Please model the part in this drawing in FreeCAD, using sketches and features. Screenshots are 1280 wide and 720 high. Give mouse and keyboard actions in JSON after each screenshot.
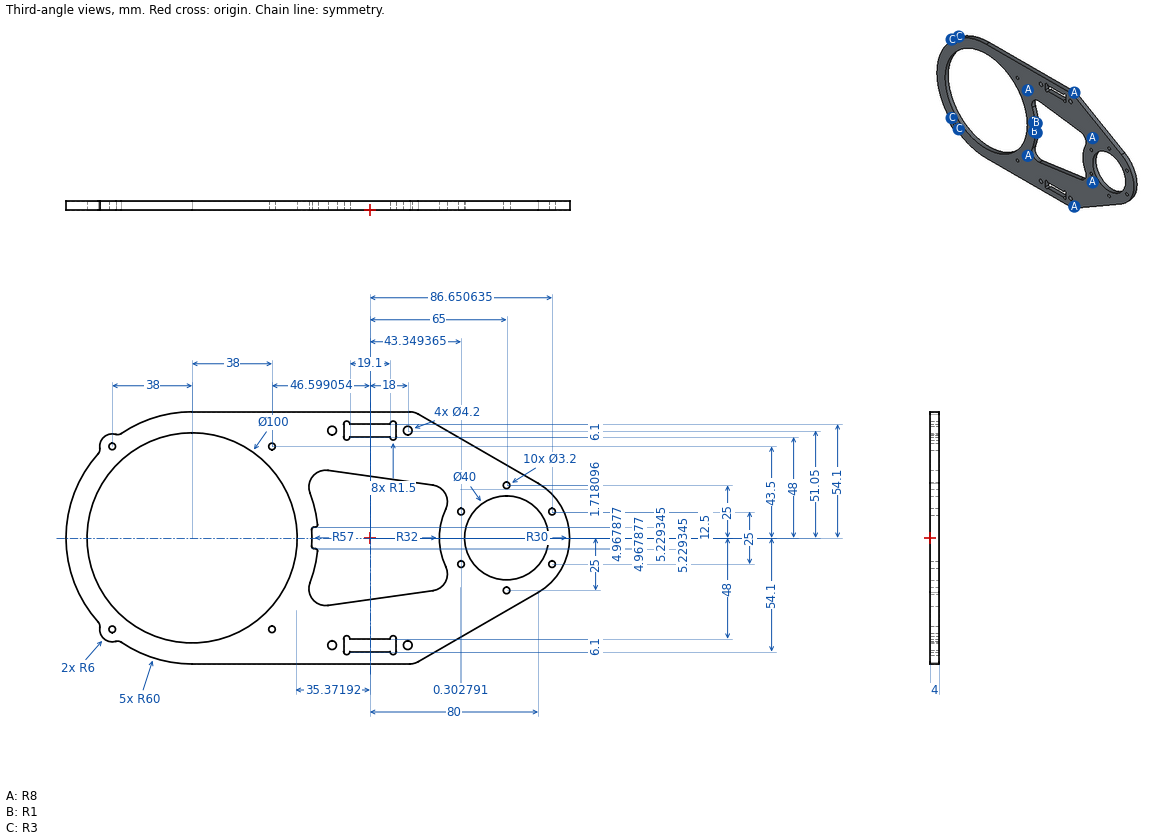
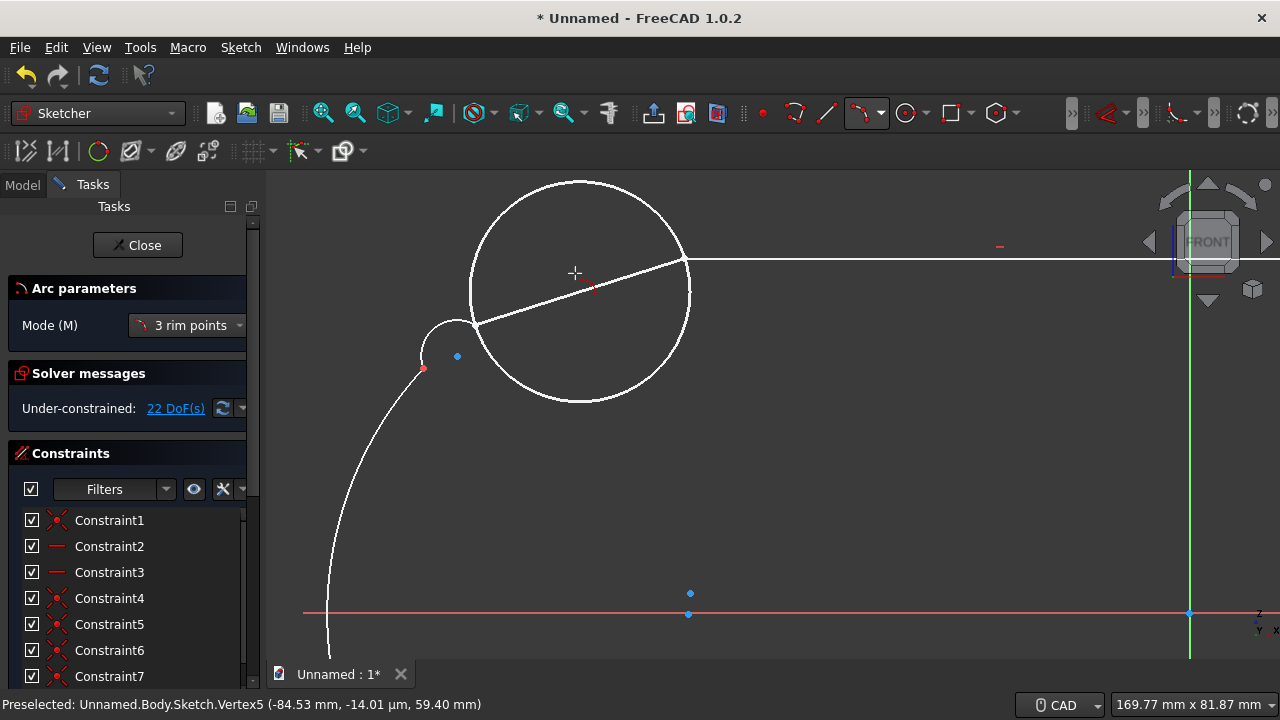
{"action": "left_click", "coordinate": [575, 272]}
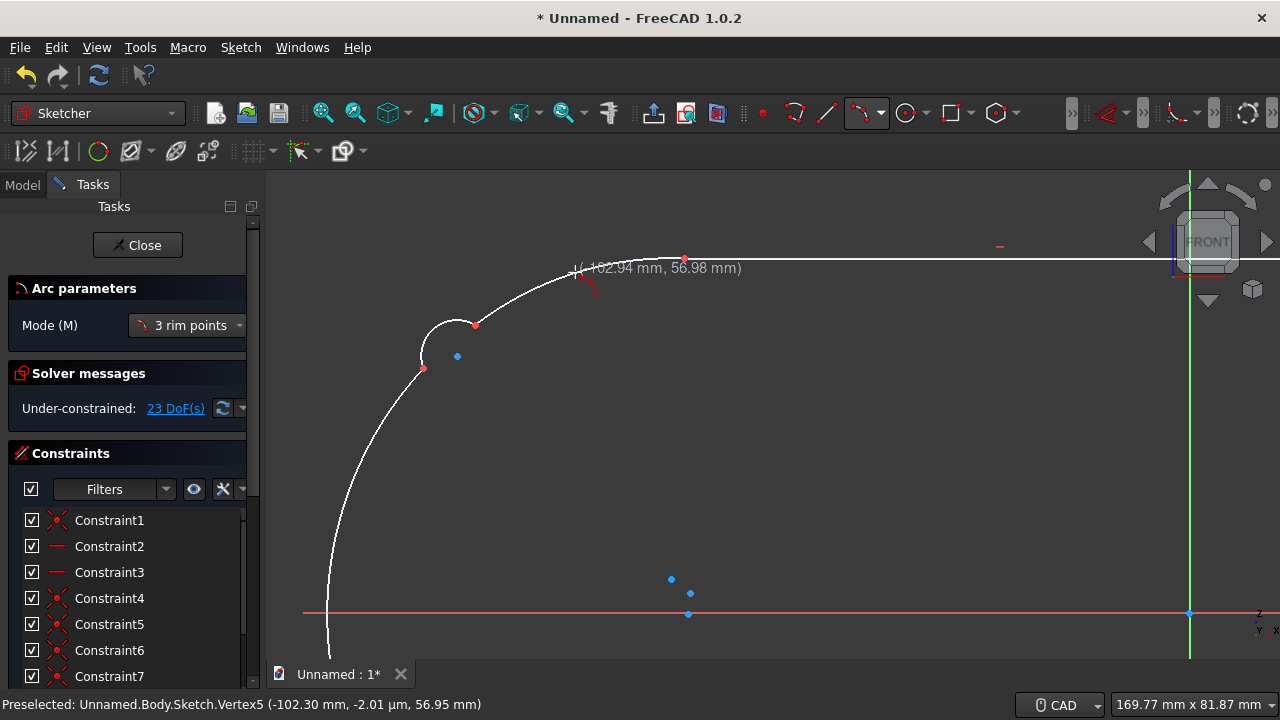
{"action": "scroll", "coordinate": [508, 299], "scroll_direction": "down", "scroll_amount": 5}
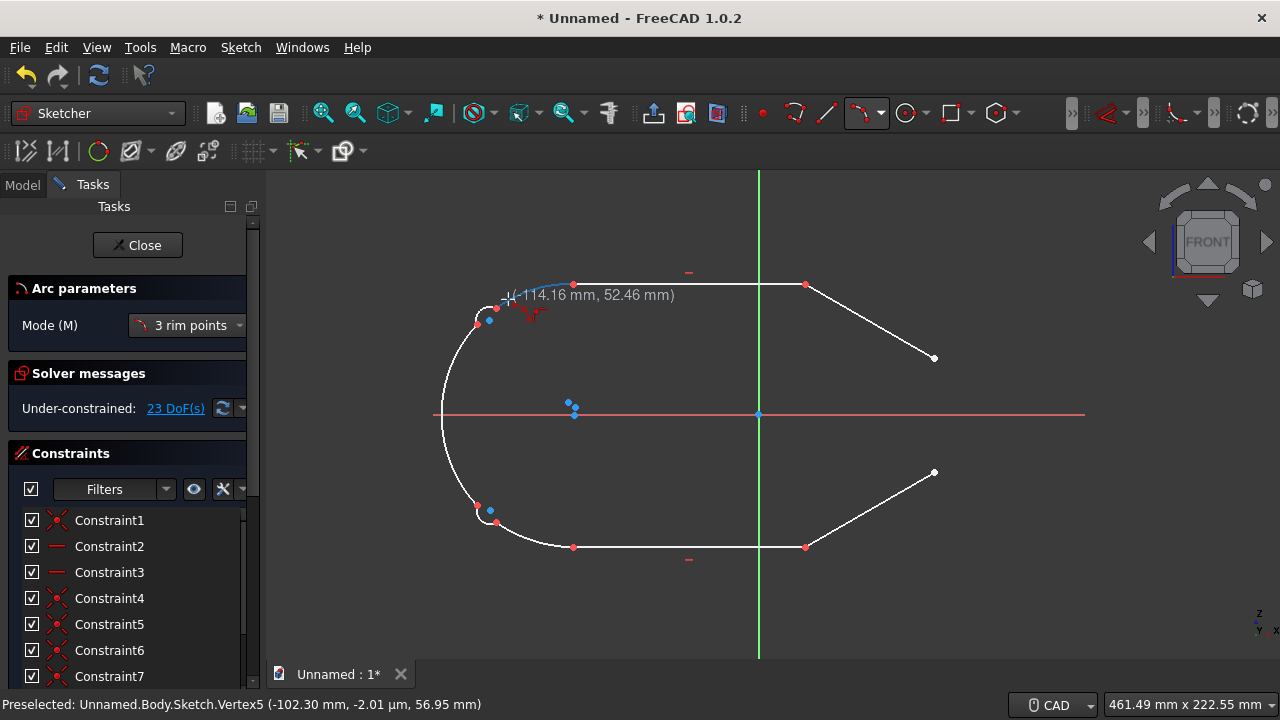
{"action": "left_click", "coordinate": [935, 359]}
{"action": "left_click", "coordinate": [935, 473]}
{"action": "left_click", "coordinate": [962, 442]}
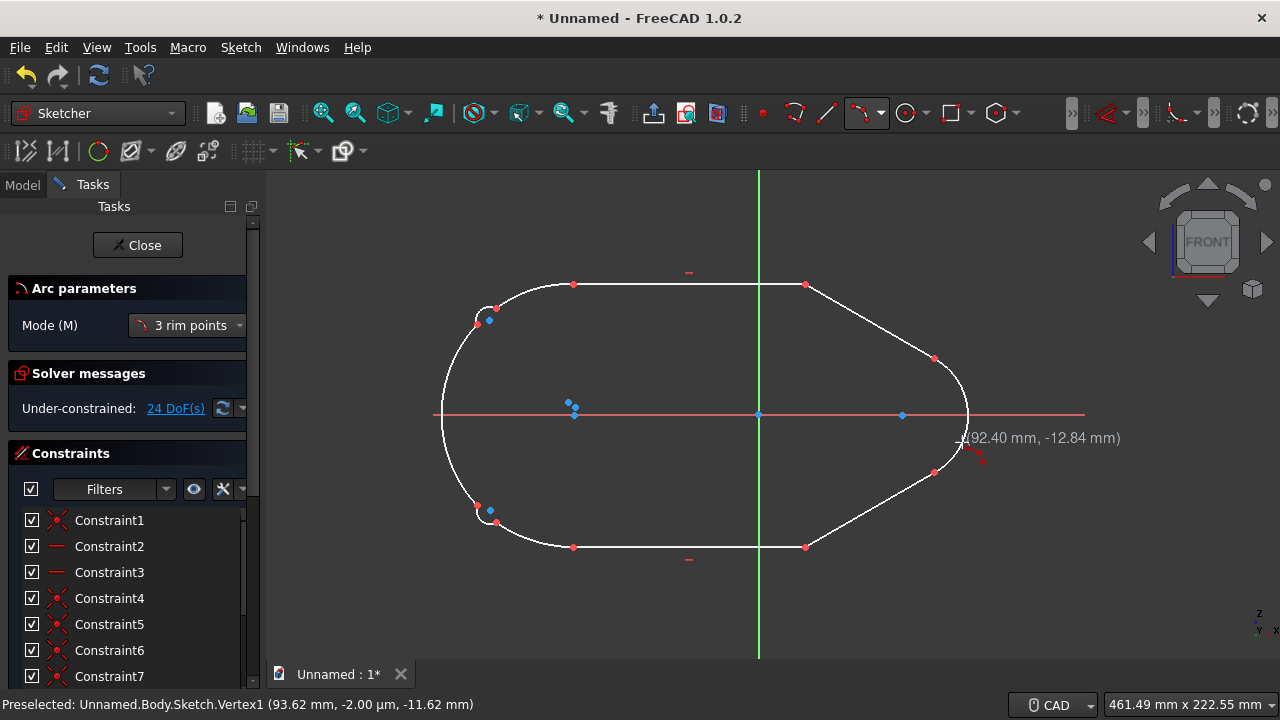
{"action": "key", "text": "g l"}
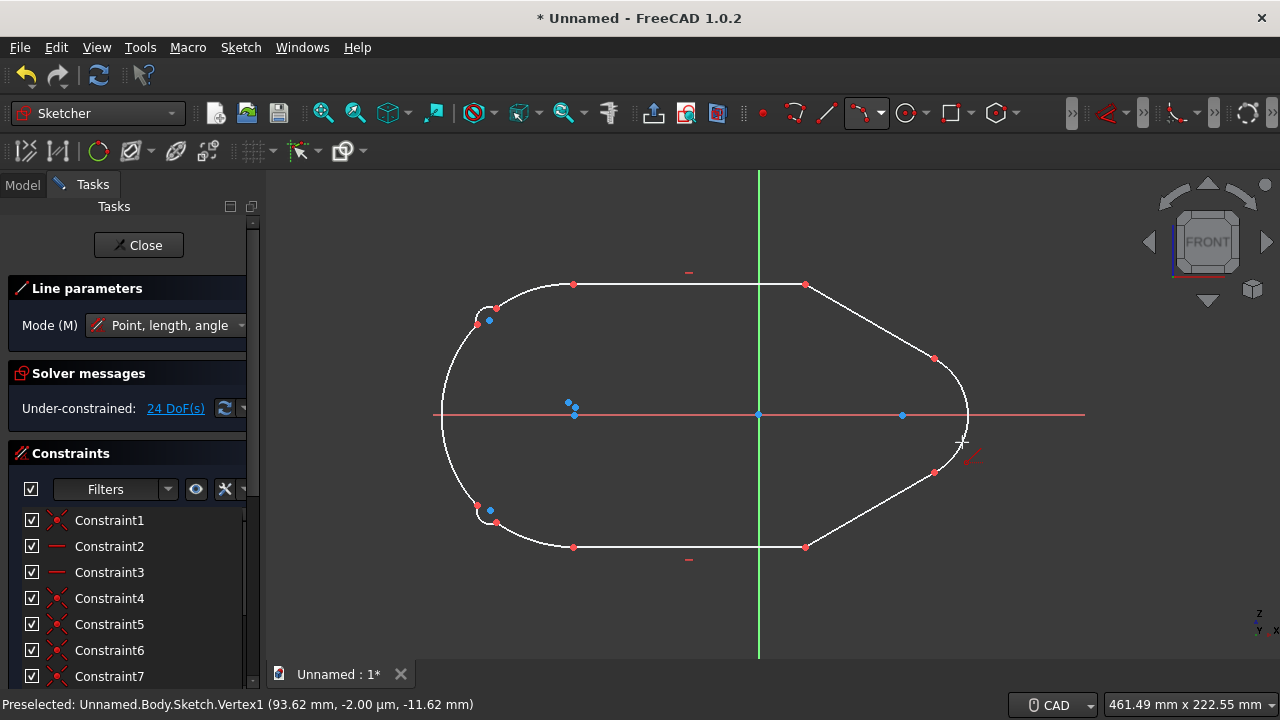
{"action": "left_click", "coordinate": [738, 309]}
{"action": "left_click", "coordinate": [780, 309]}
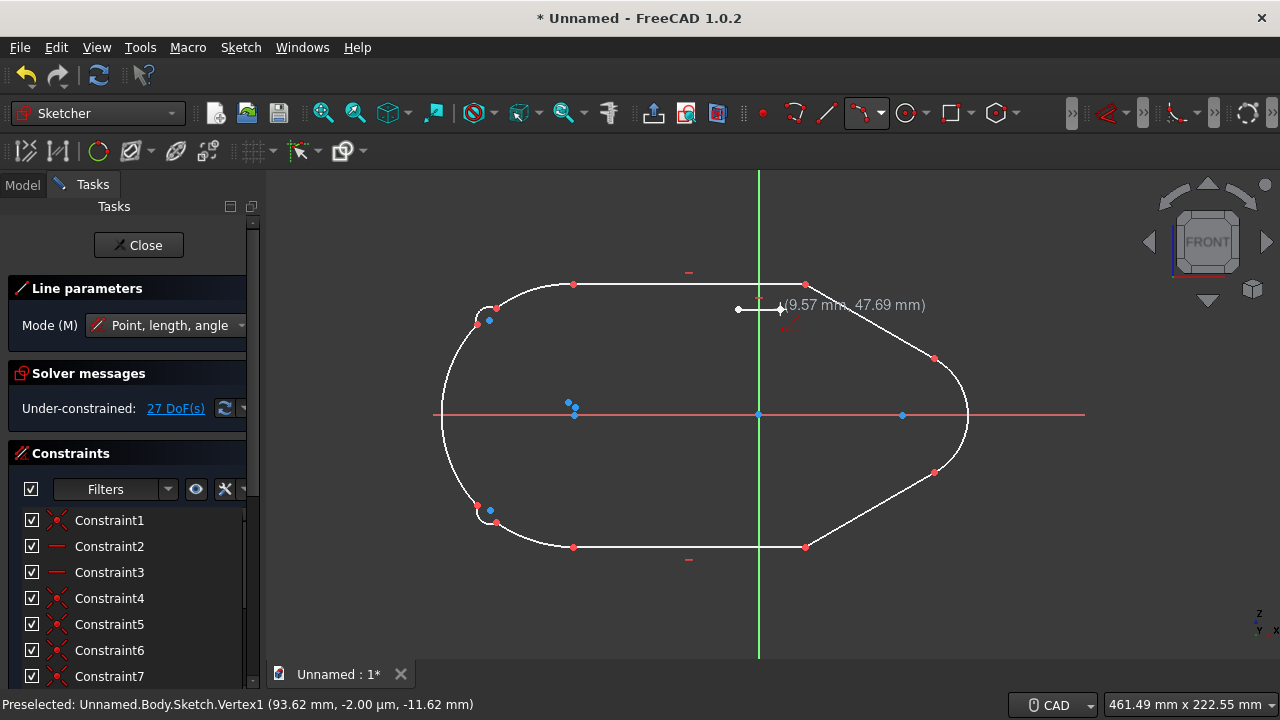
{"action": "scroll", "coordinate": [787, 309], "scroll_direction": "up", "scroll_amount": 5}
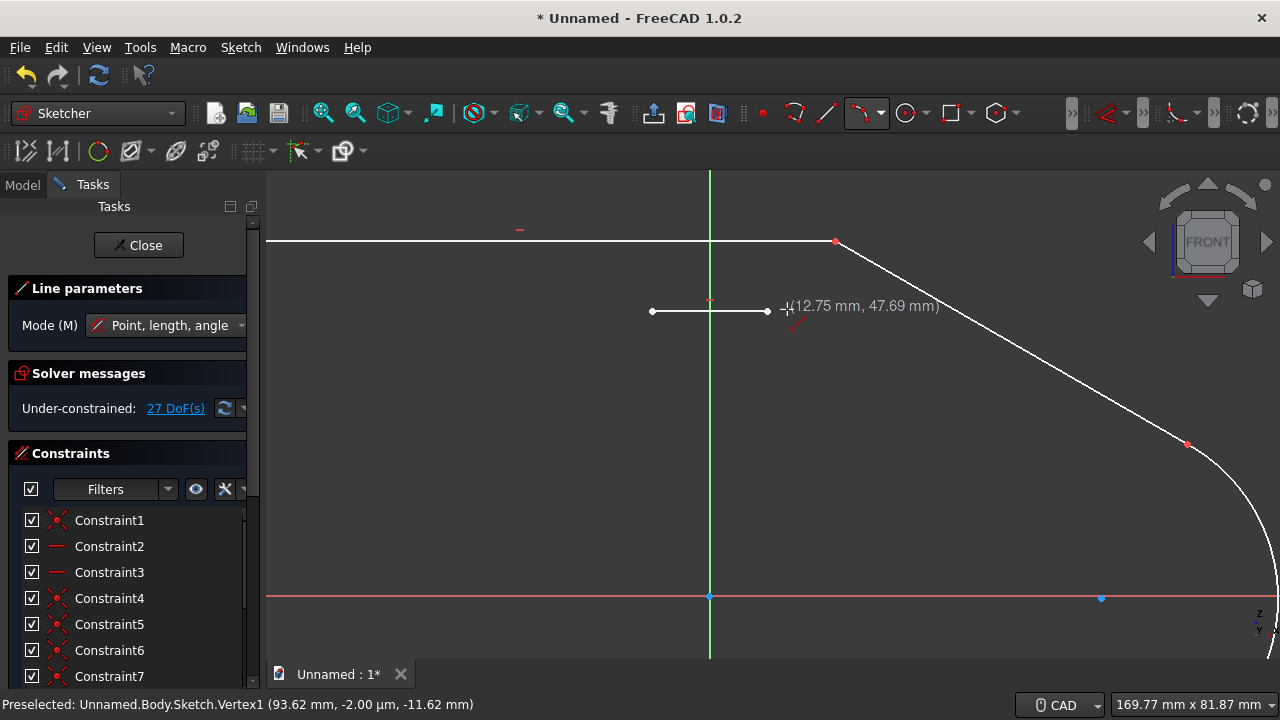
{"action": "left_click", "coordinate": [785, 309]}
{"action": "left_click", "coordinate": [785, 273]}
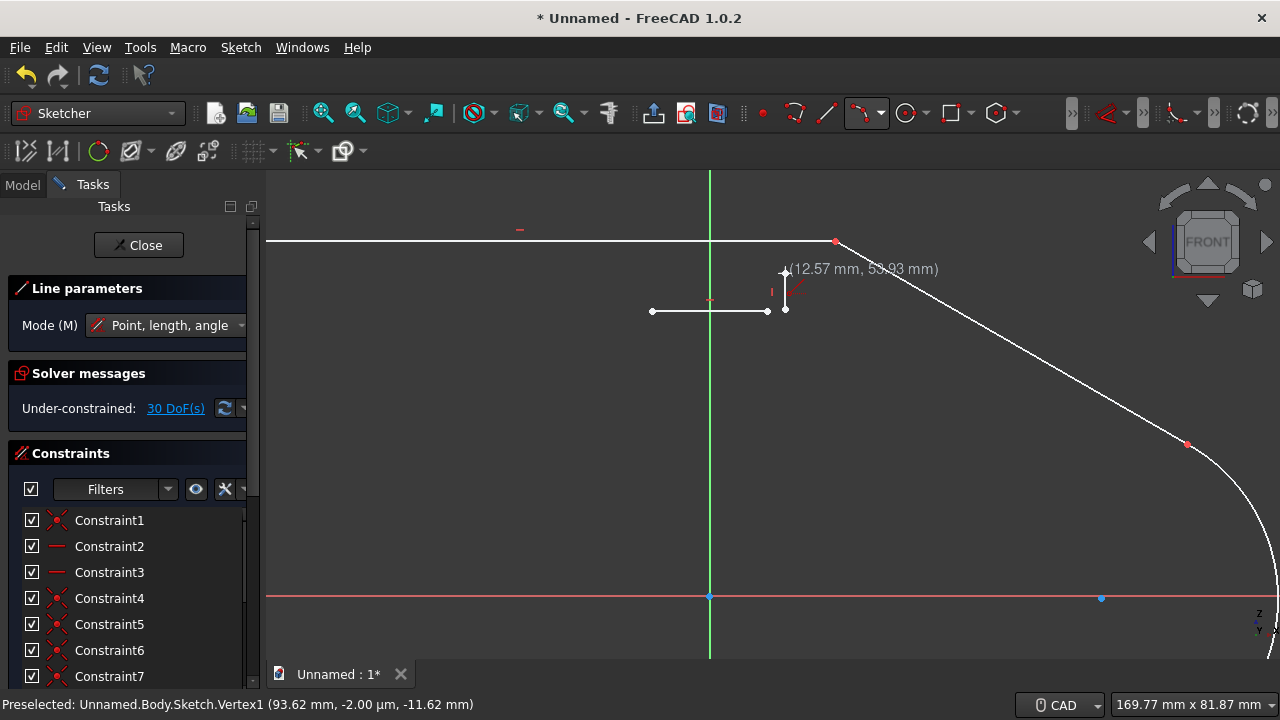
{"action": "left_click", "coordinate": [767, 273]}
{"action": "left_click", "coordinate": [653, 273]}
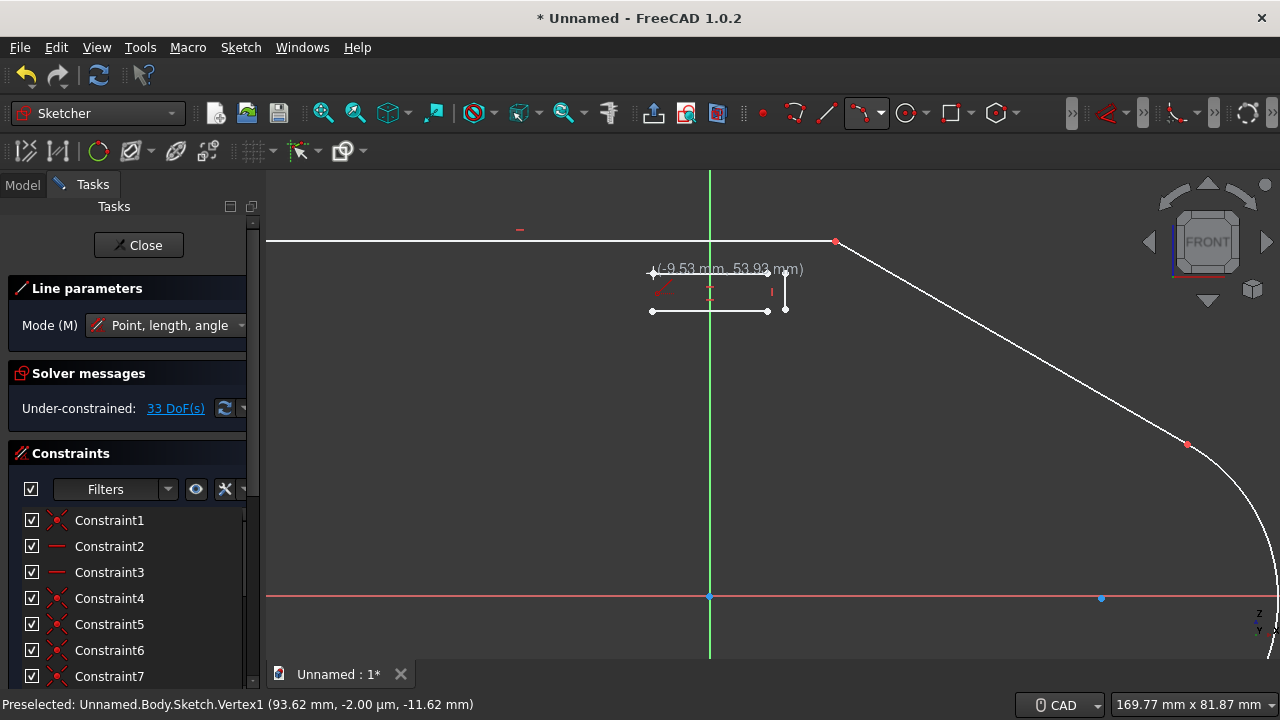
{"action": "left_click", "coordinate": [635, 273]}
{"action": "left_click", "coordinate": [635, 309]}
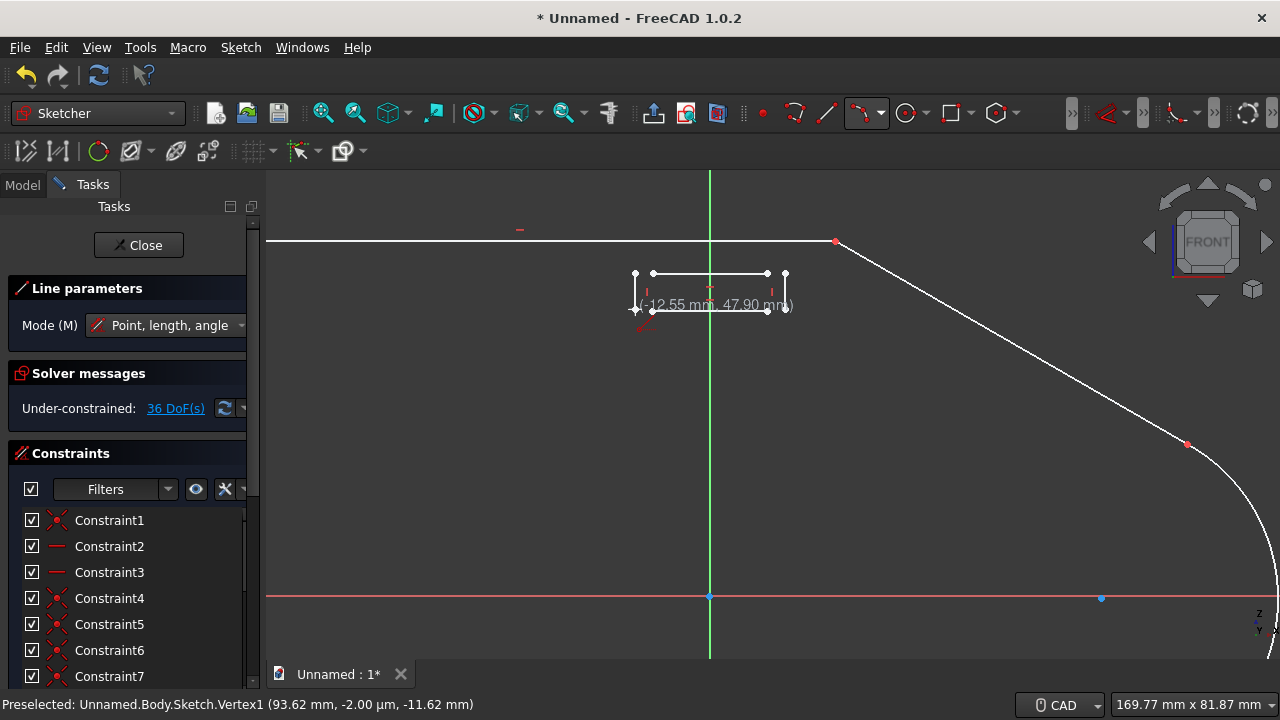
{"action": "key", "text": "g 3 a"}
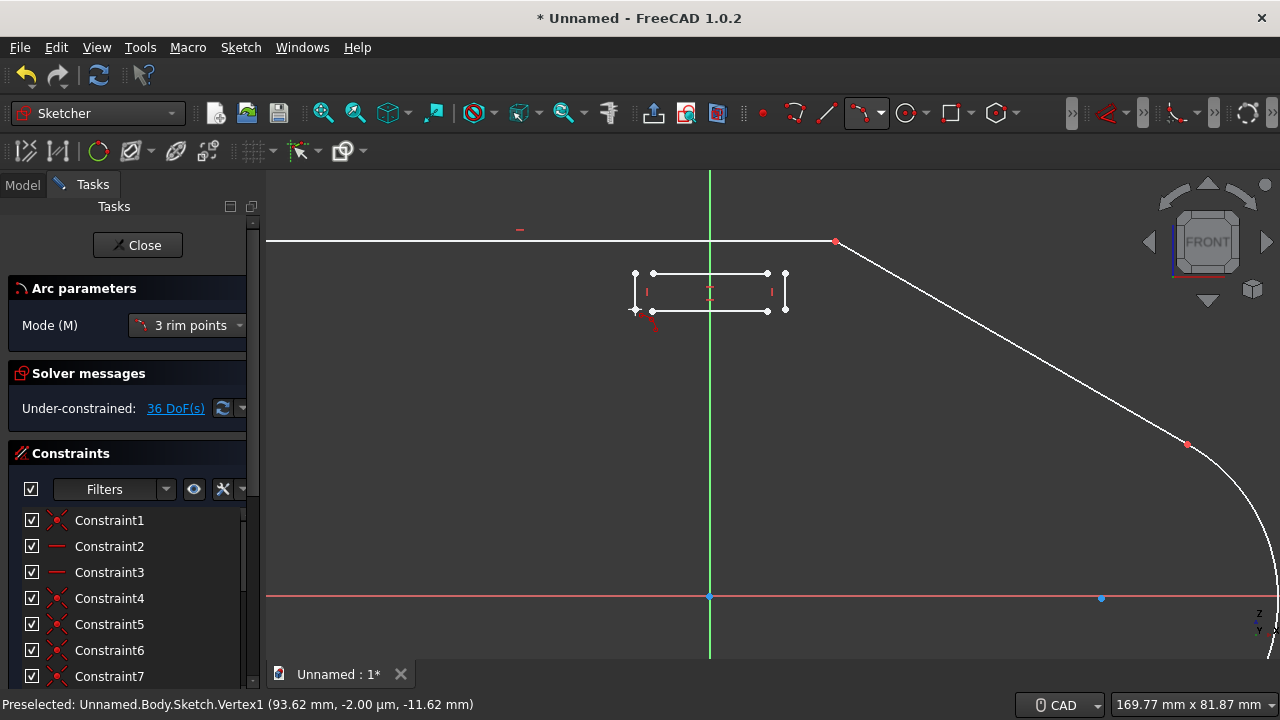
{"action": "left_click", "coordinate": [767, 311]}
{"action": "left_click", "coordinate": [785, 310]}